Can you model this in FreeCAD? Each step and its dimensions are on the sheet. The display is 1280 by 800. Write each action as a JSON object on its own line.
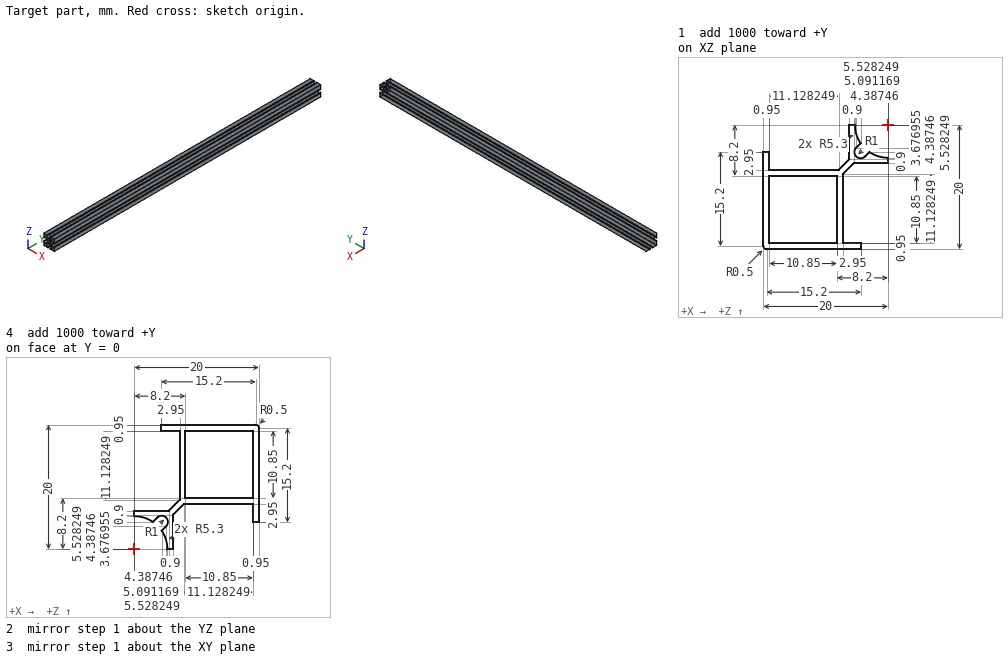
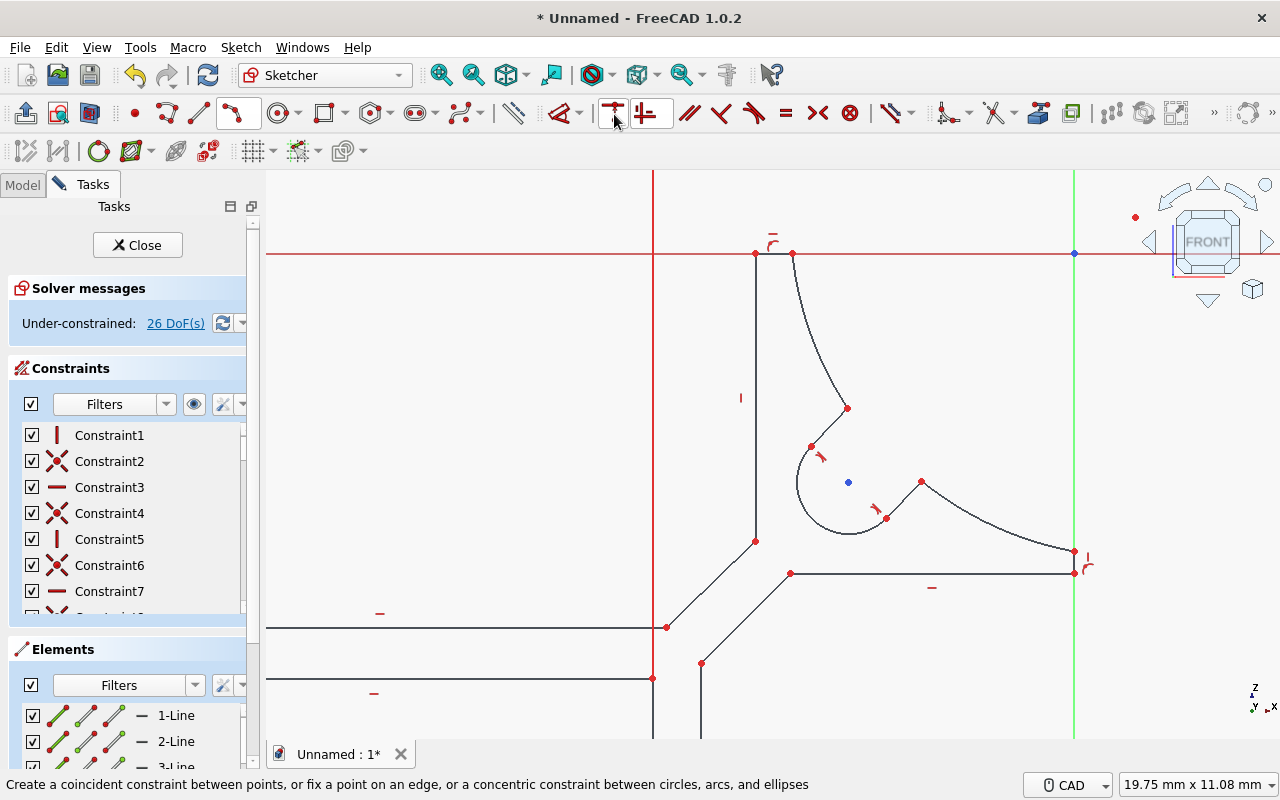
{"action": "left_click_drag", "start_coordinate": [1064, 208], "coordinate": [1145, 264]}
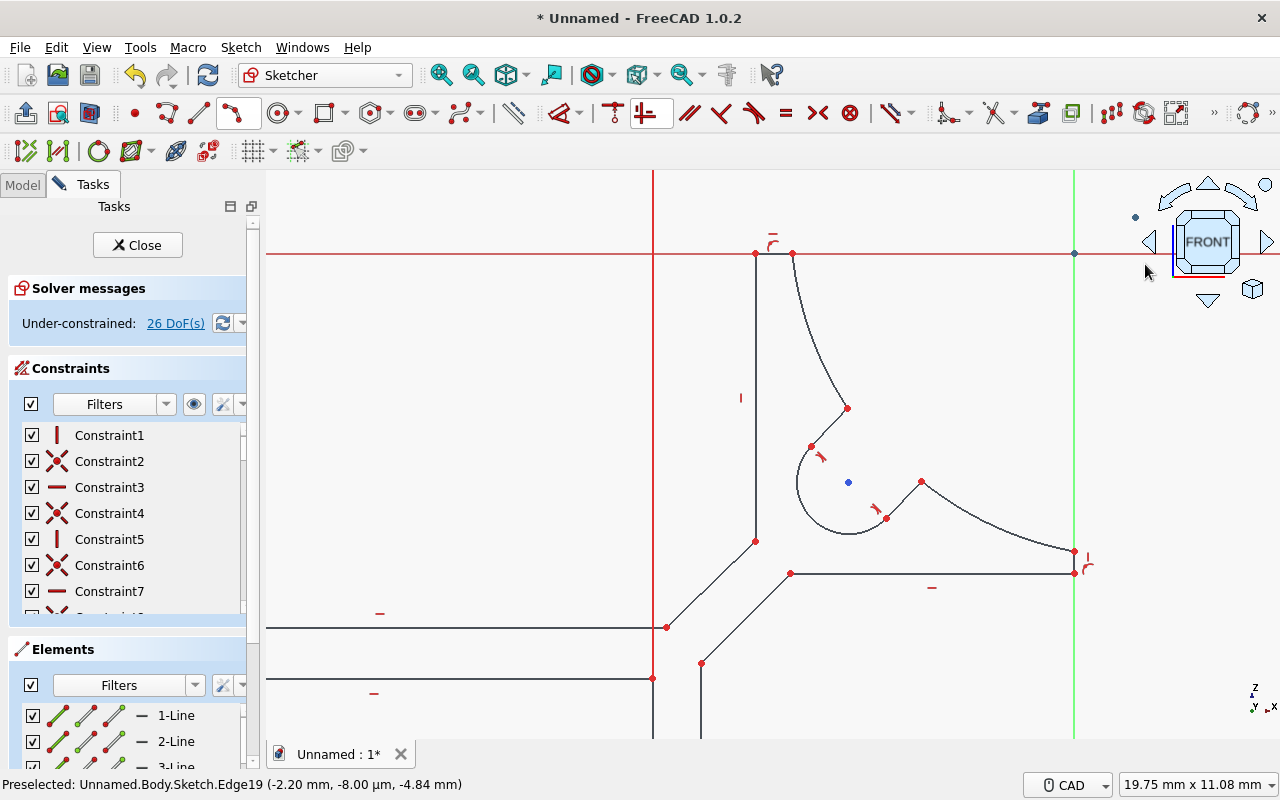
{"action": "key", "text": "c"}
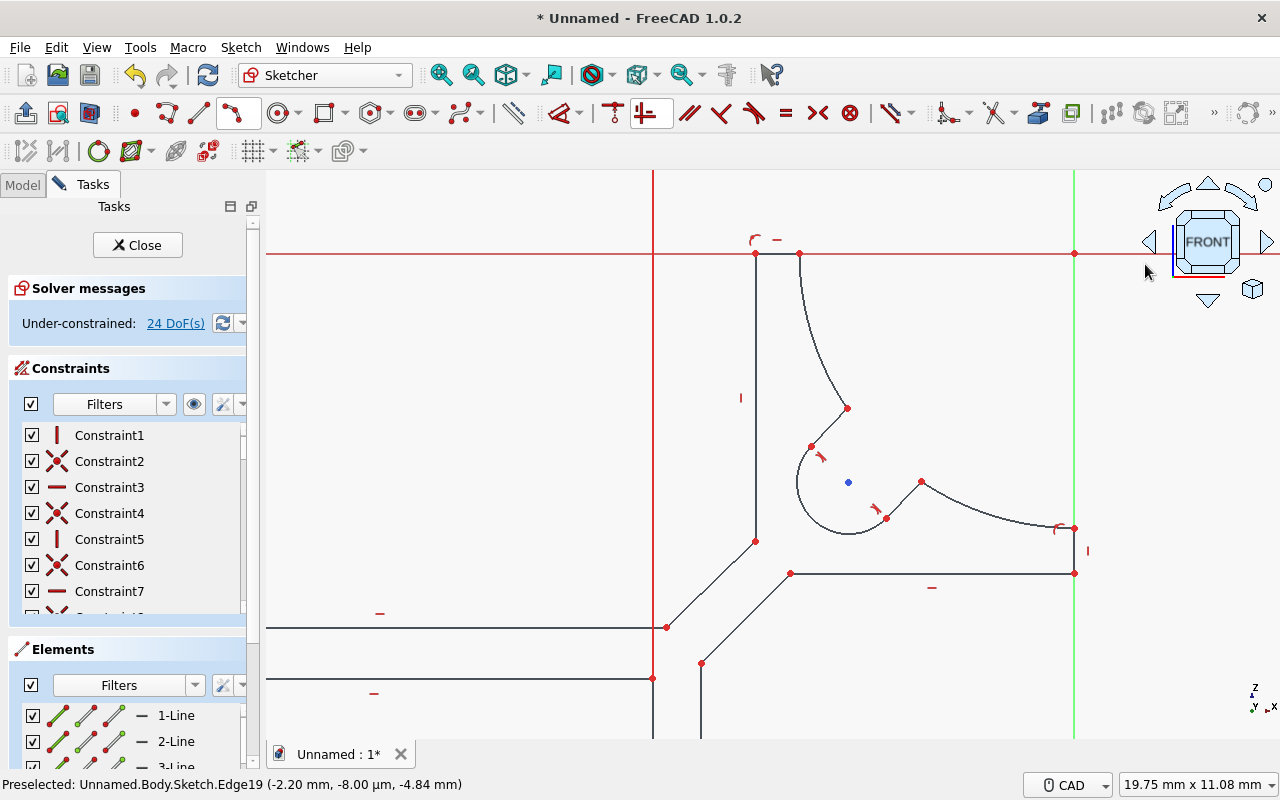
{"action": "left_click", "coordinate": [804, 303]}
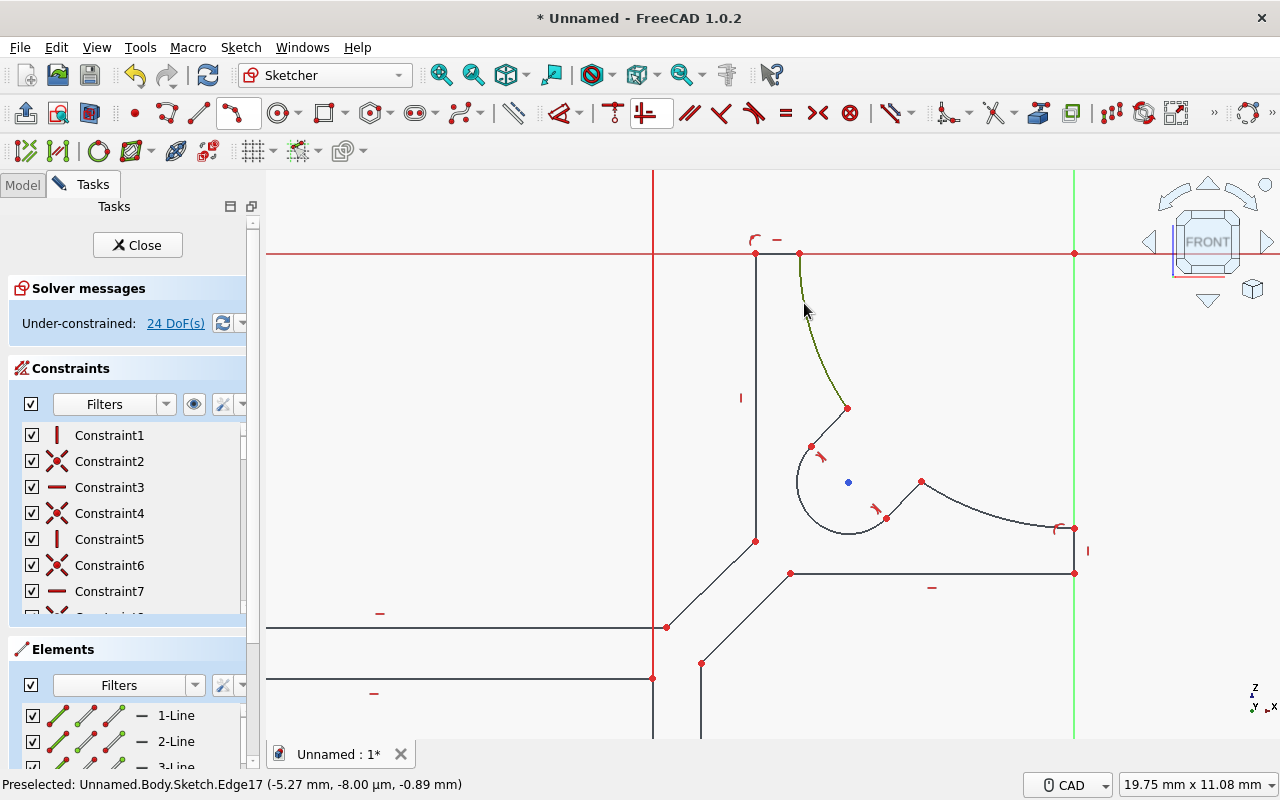
{"action": "left_click", "coordinate": [964, 505]}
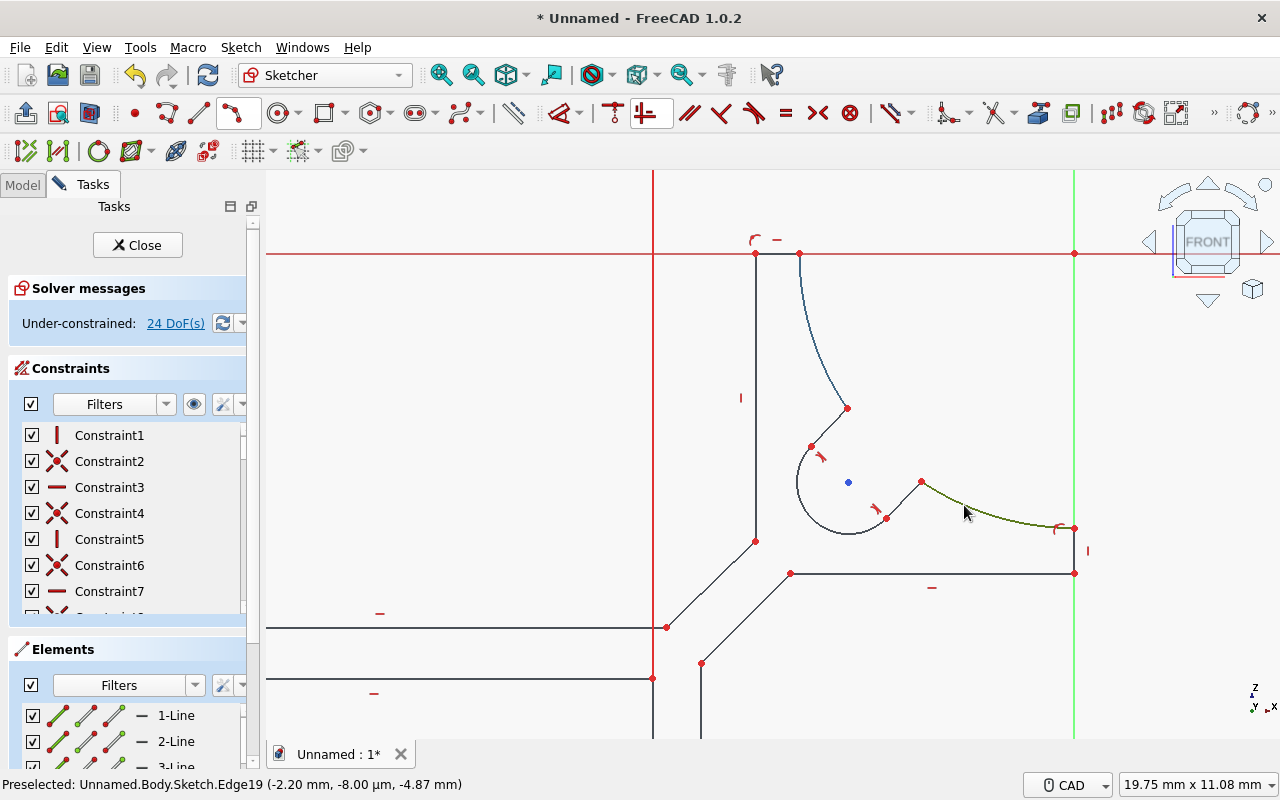
{"action": "left_click", "coordinate": [786, 114]}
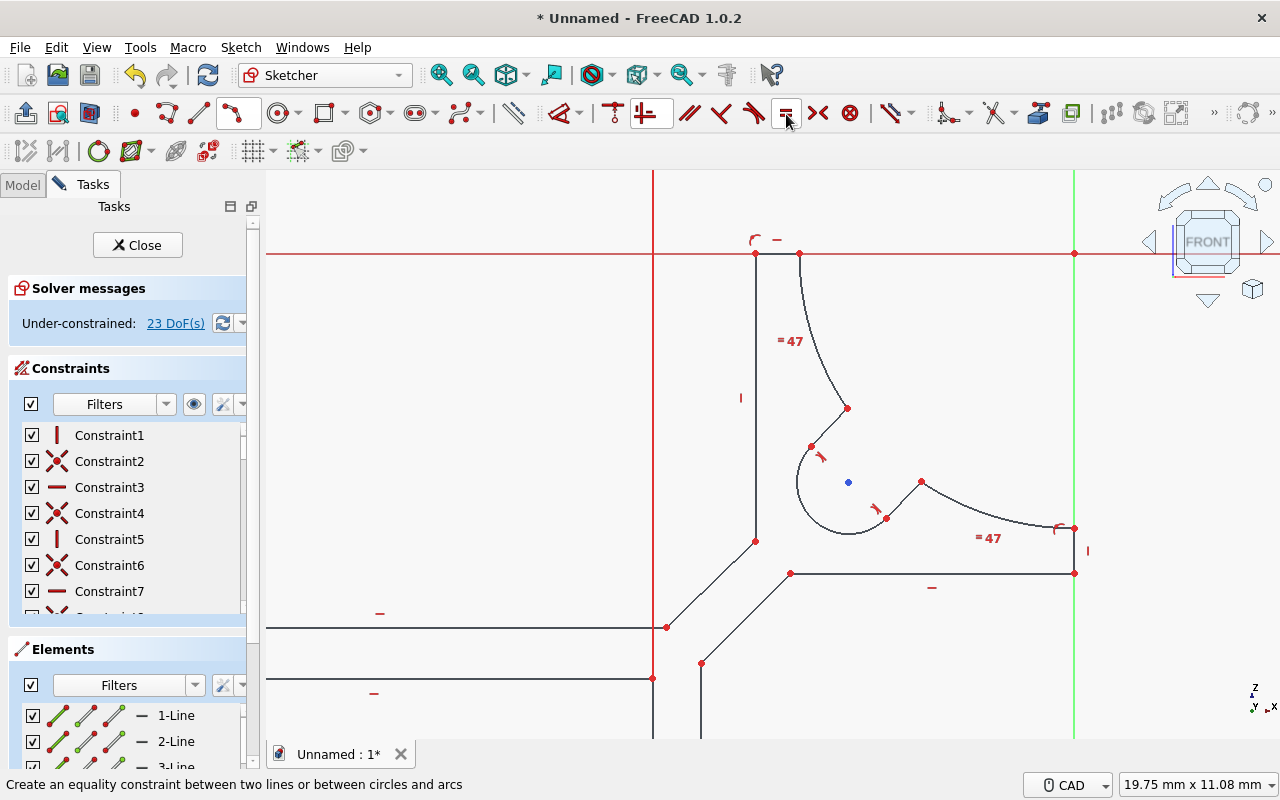
{"action": "left_click", "coordinate": [560, 114]}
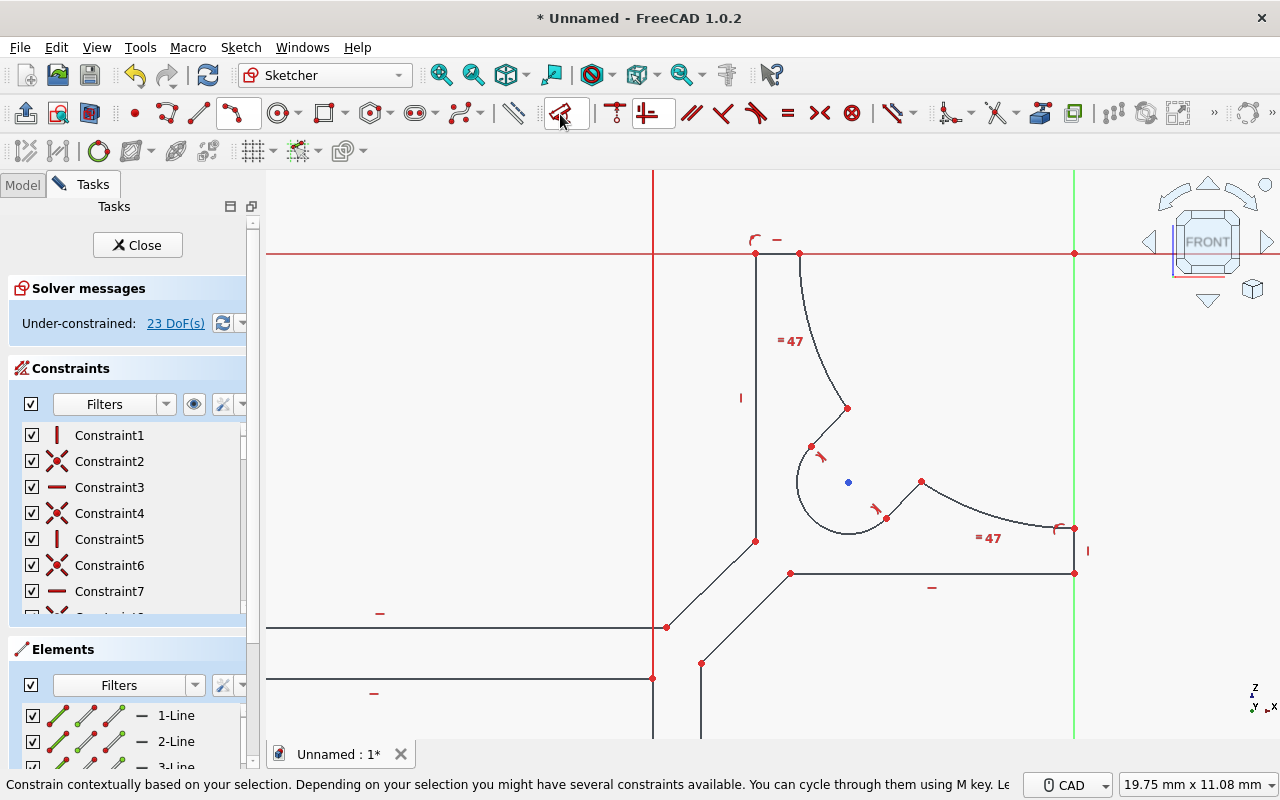
{"action": "left_click", "coordinate": [804, 303]}
{"action": "left_click", "coordinate": [773, 309]}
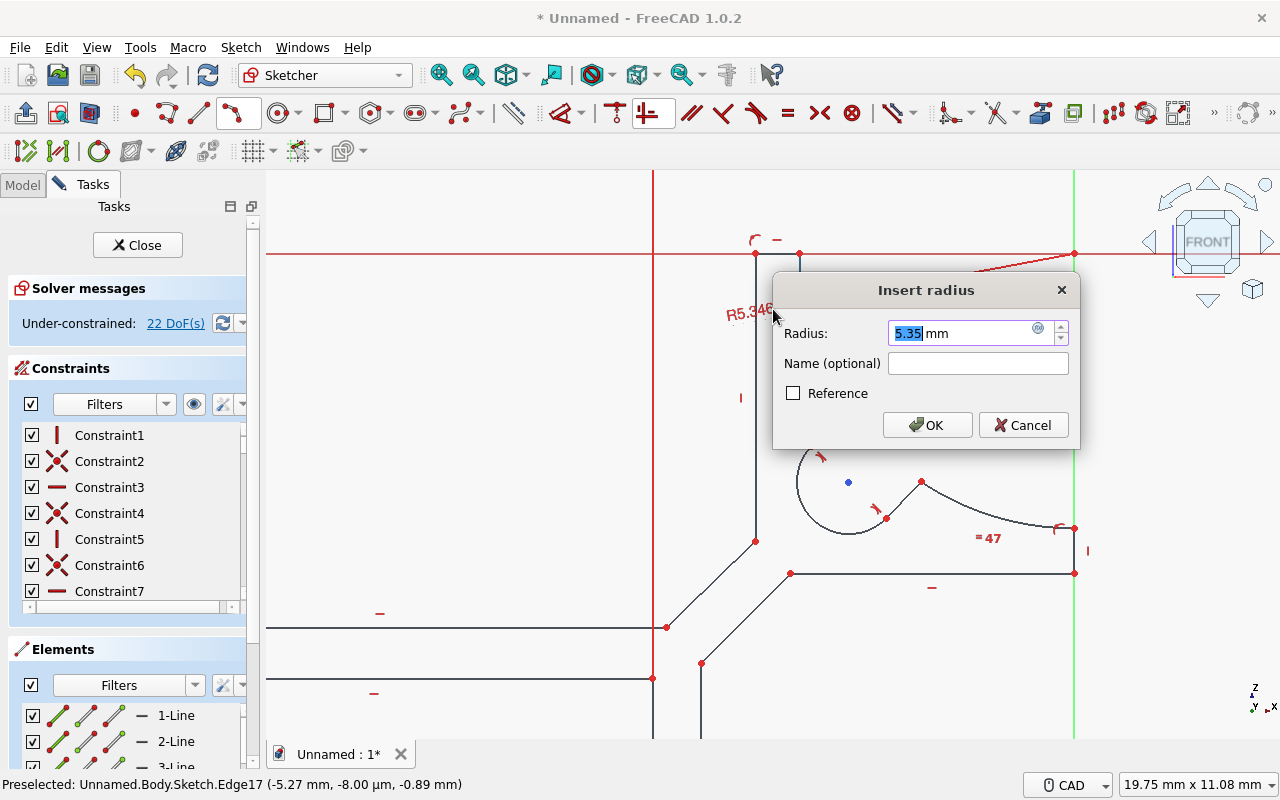
{"action": "type", "text": "5.3"}
{"action": "key", "text": "Return"}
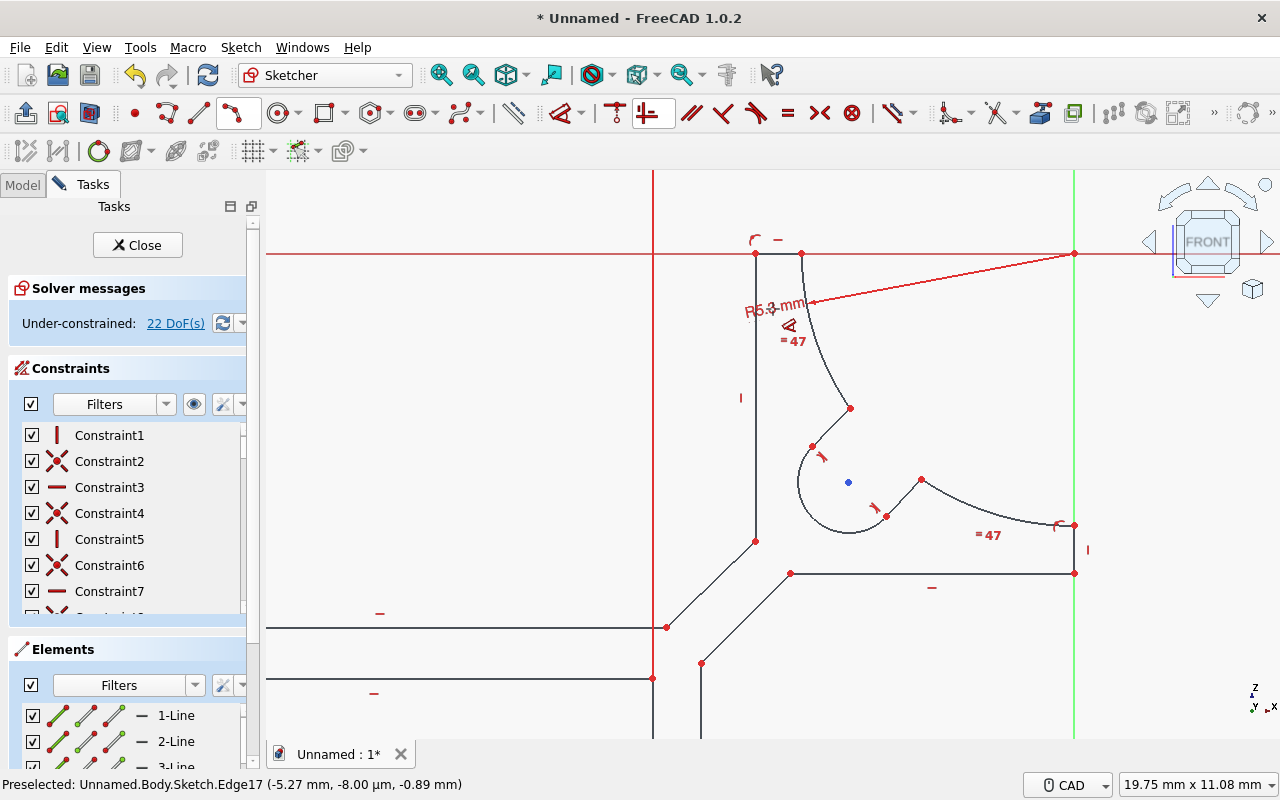
{"action": "left_click", "coordinate": [799, 491]}
{"action": "left_click", "coordinate": [771, 456]}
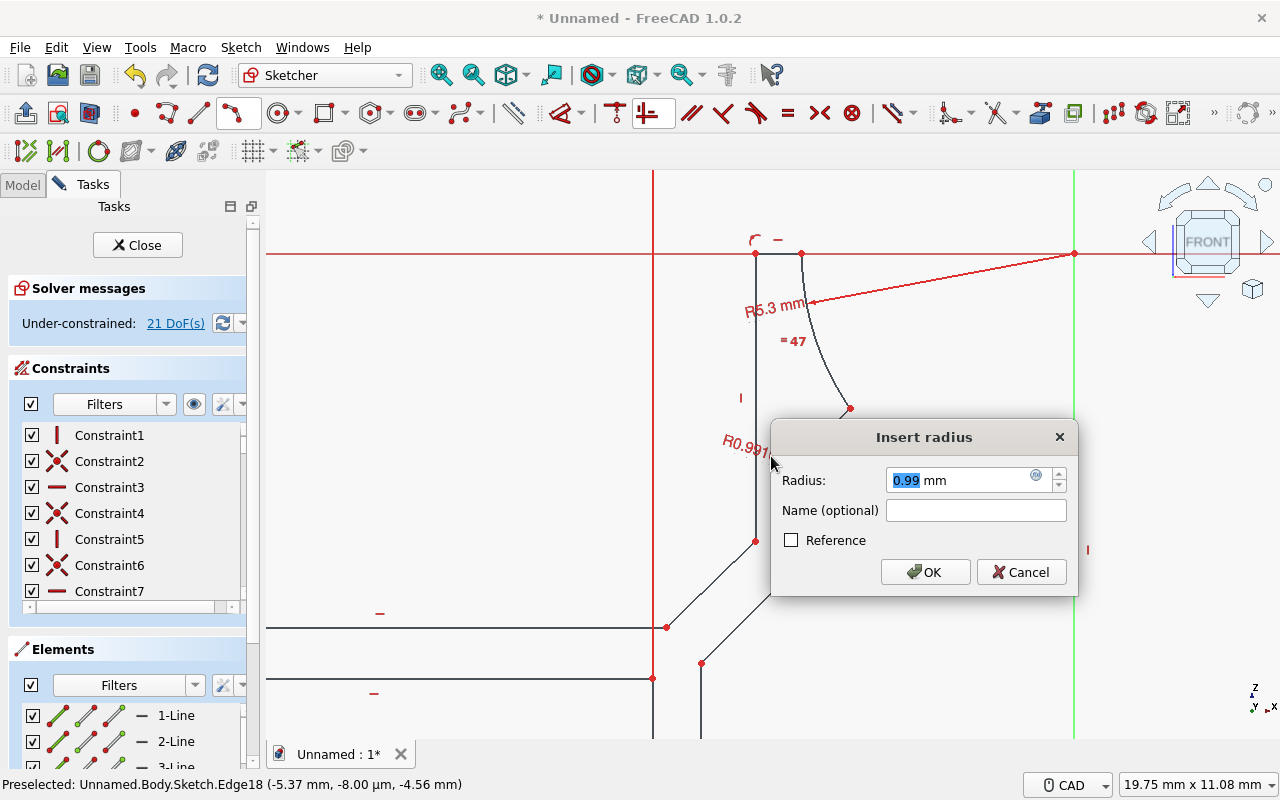
{"action": "type", "text": "1"}
{"action": "key", "text": "Return"}